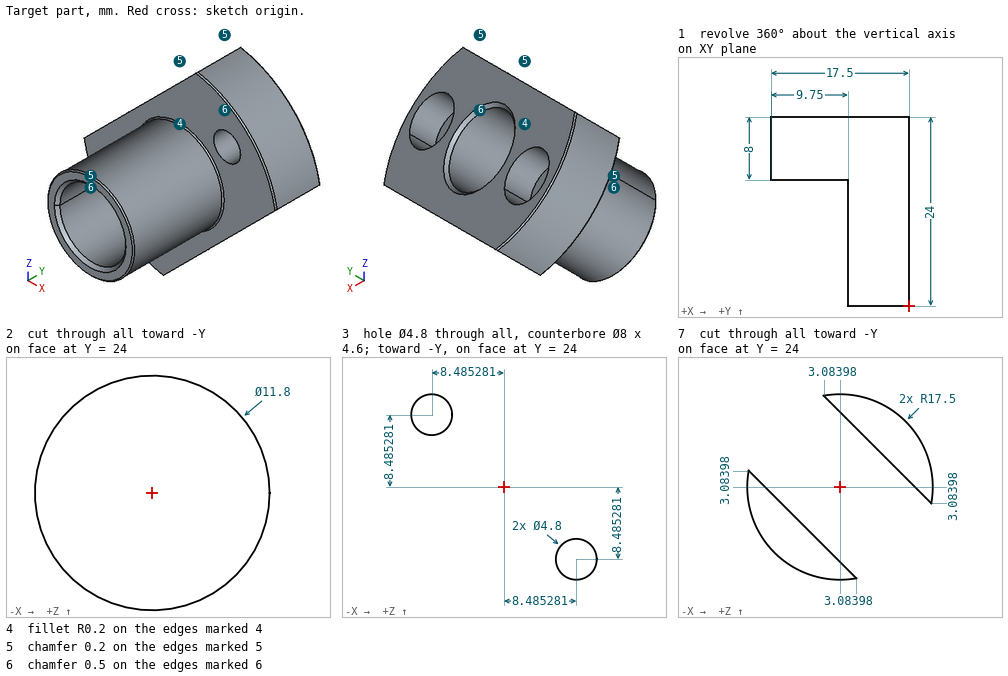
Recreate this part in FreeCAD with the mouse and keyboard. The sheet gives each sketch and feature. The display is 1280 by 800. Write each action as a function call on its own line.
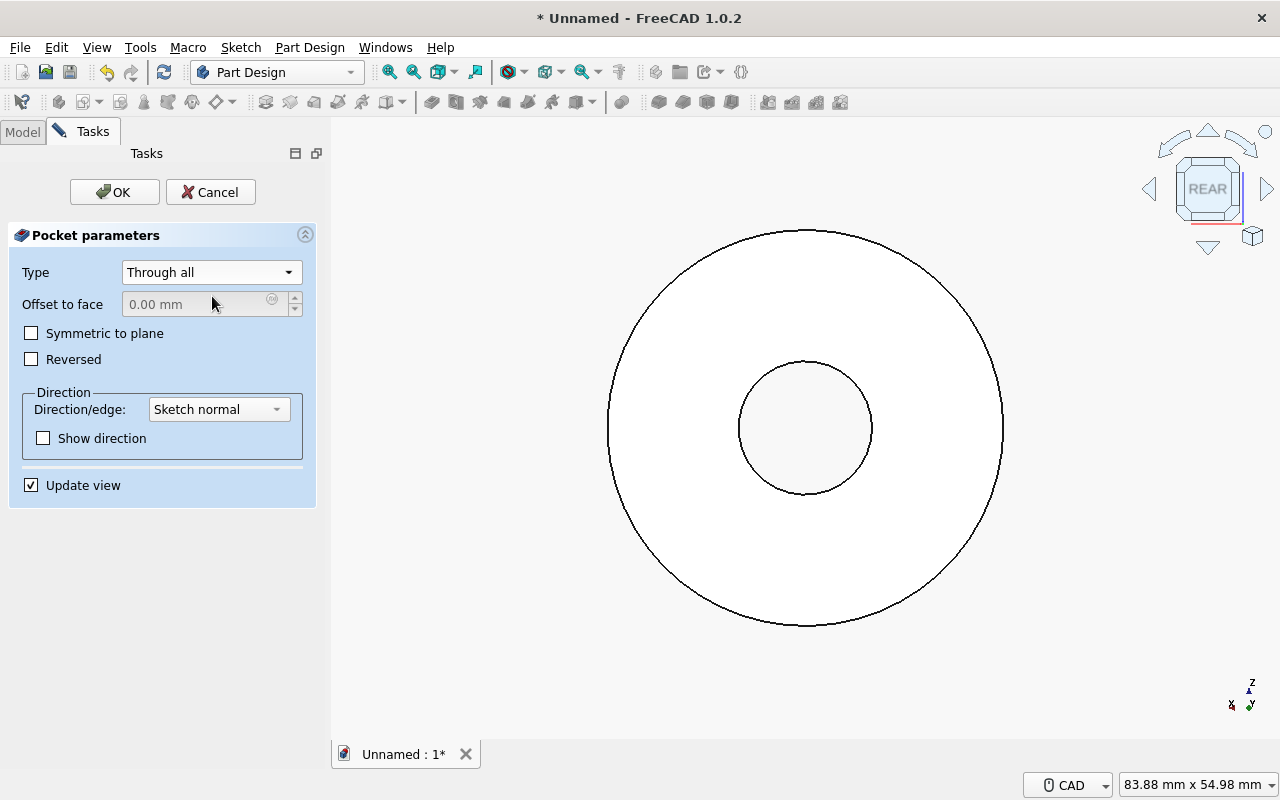
click(115, 192)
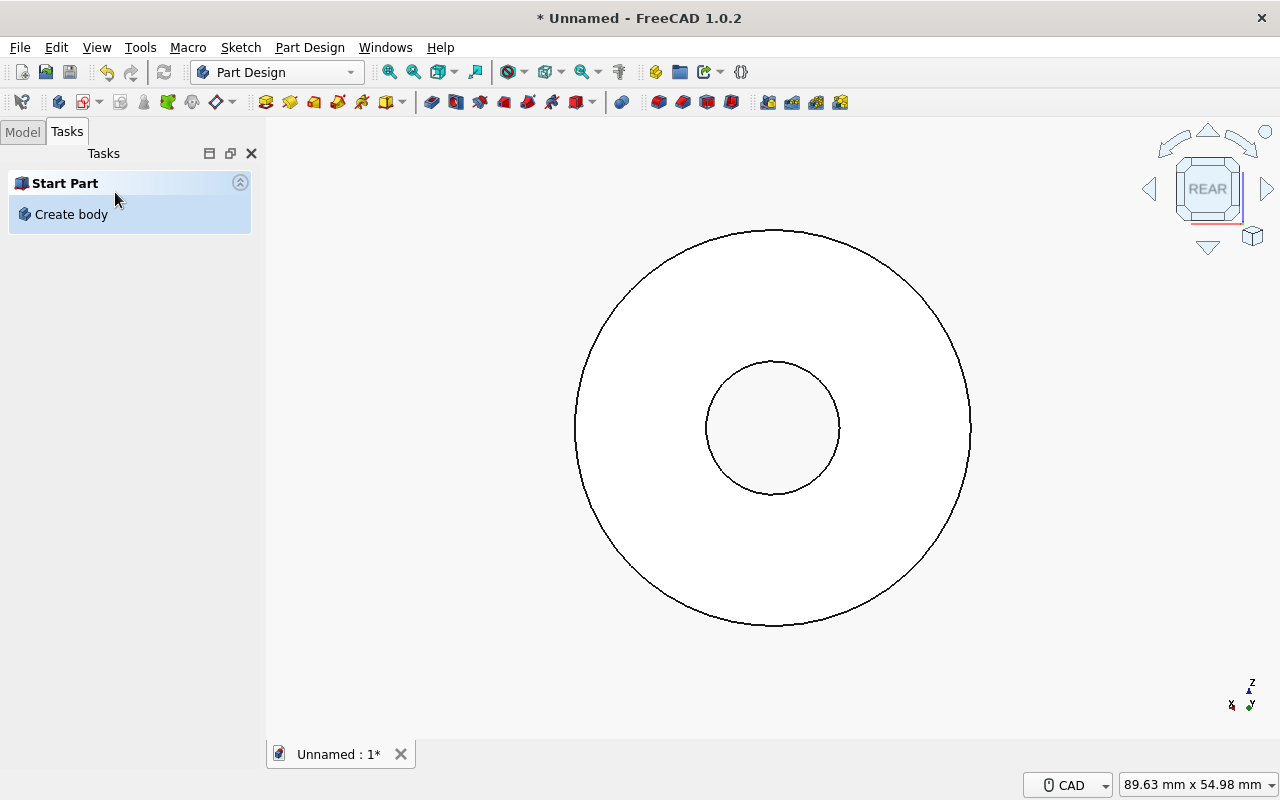
click(829, 540)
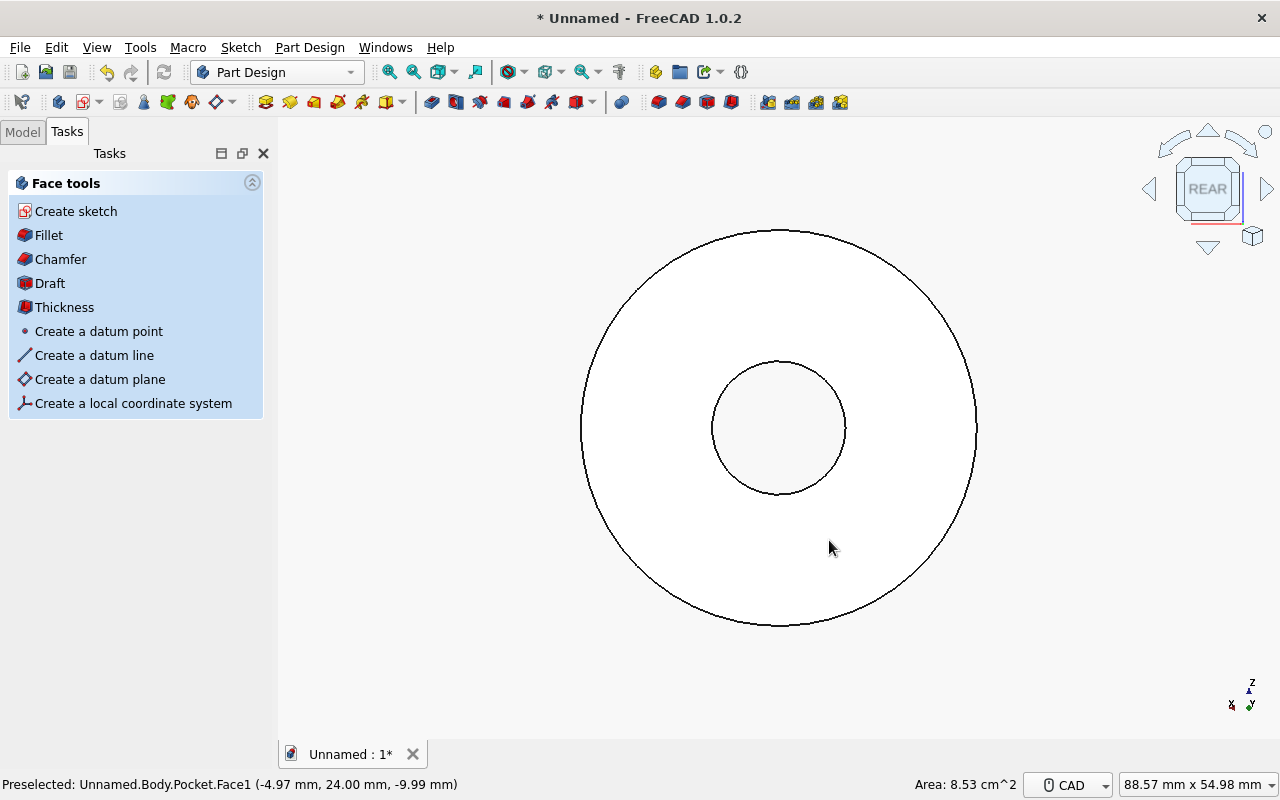
click(84, 102)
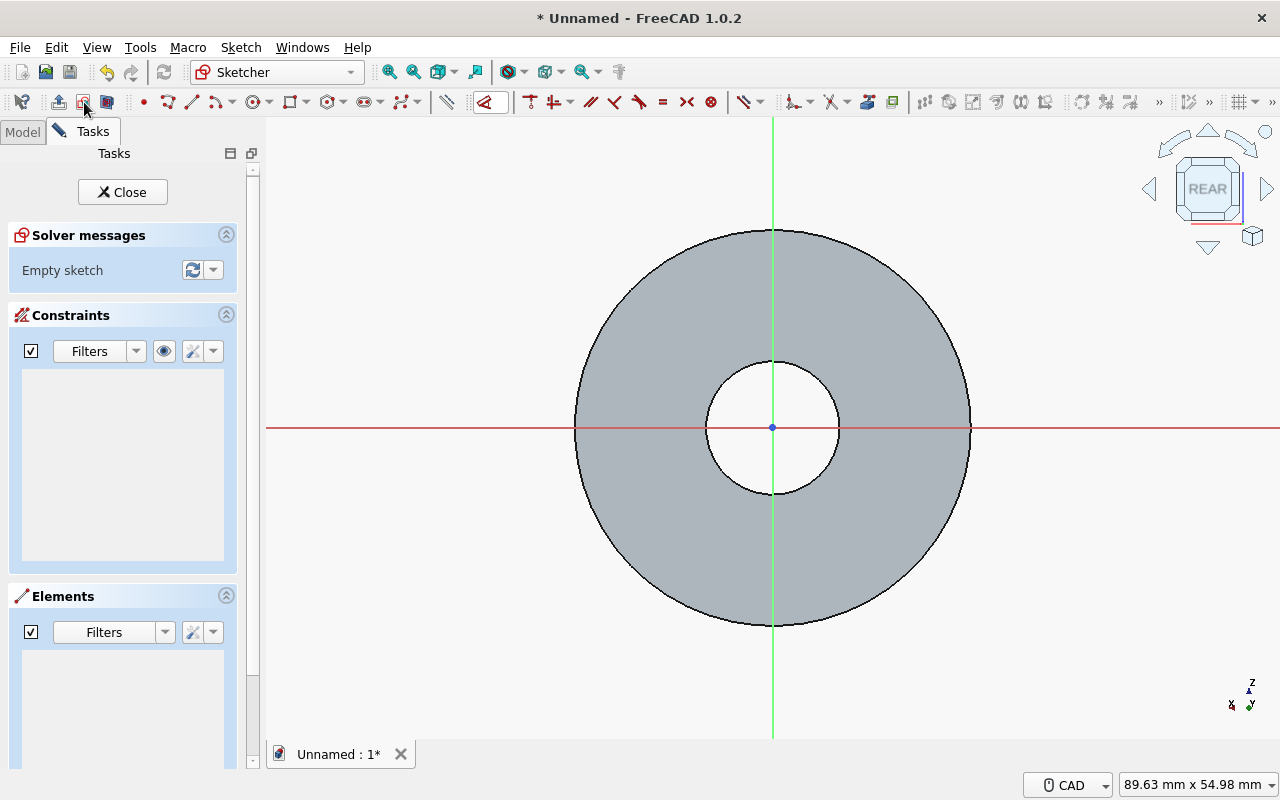
scroll(912, 428, up, 2)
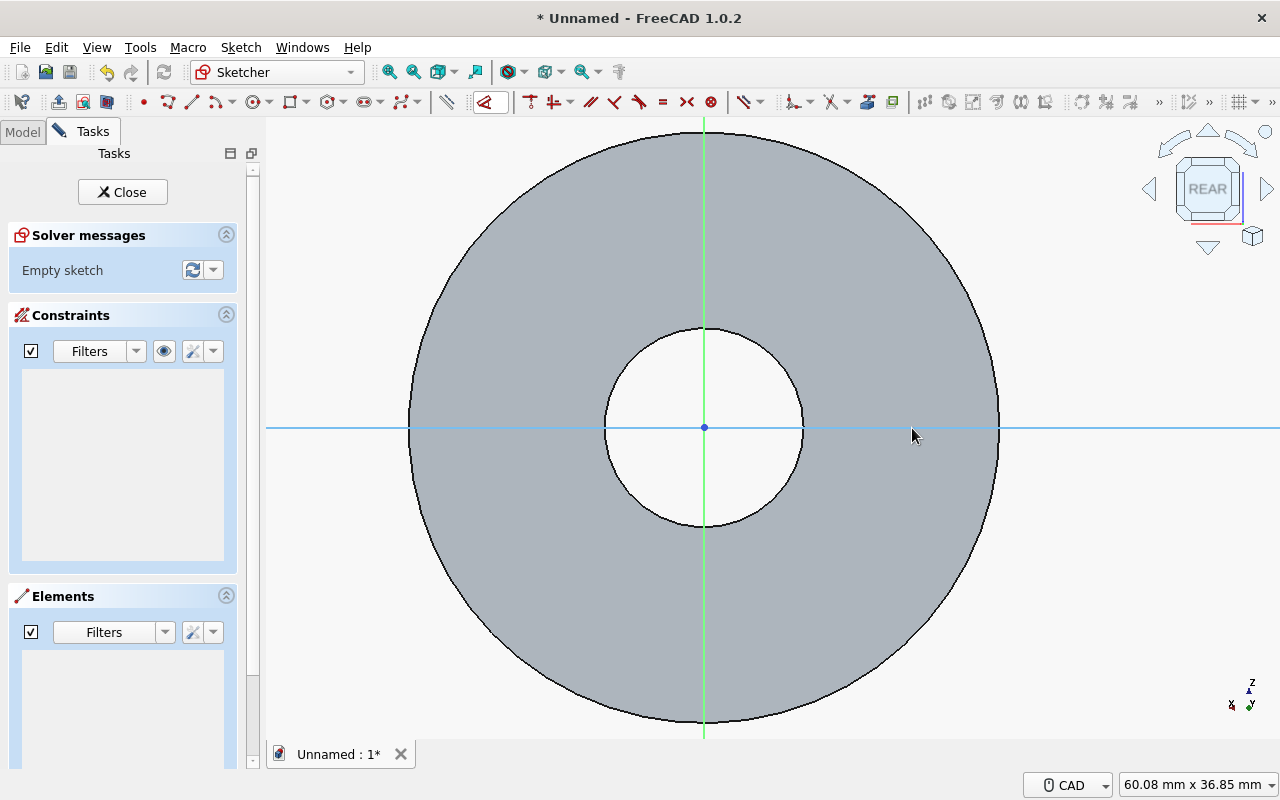
key(g)
key(c)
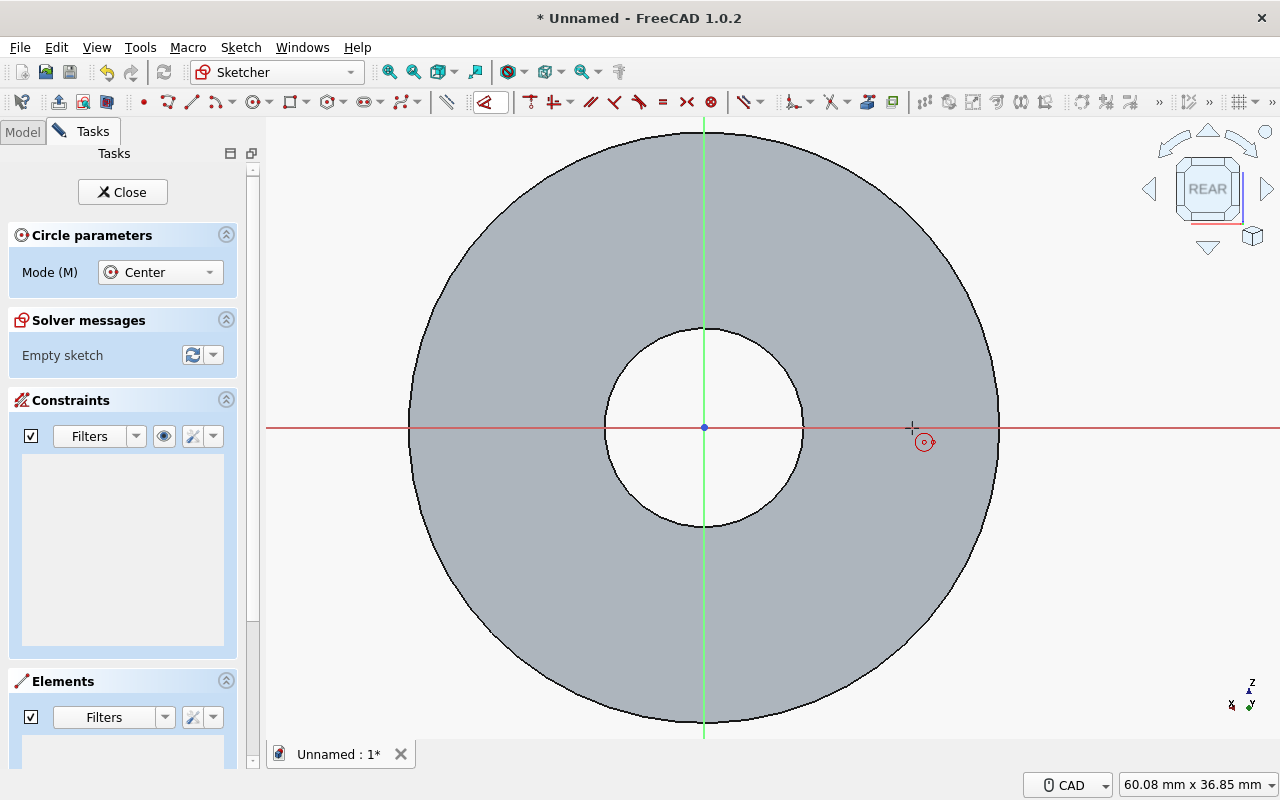
click(847, 571)
click(876, 542)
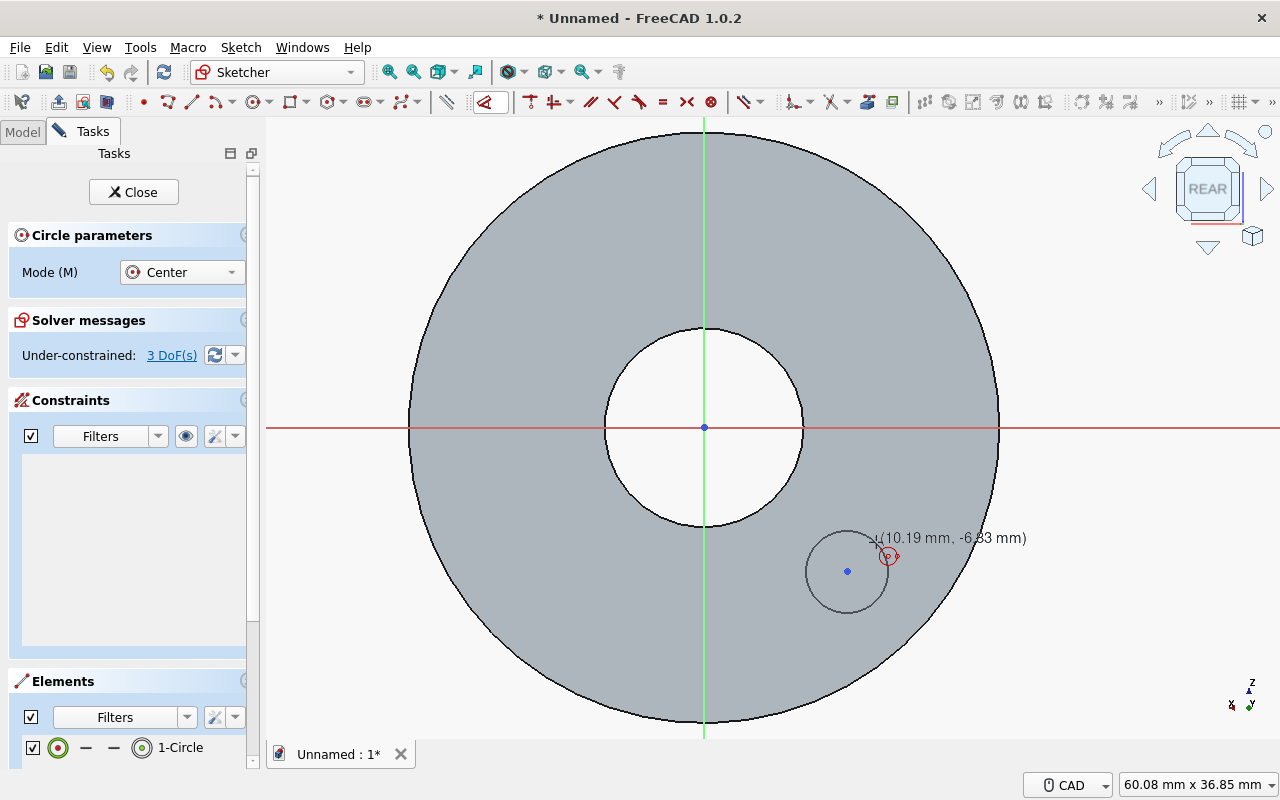
click(561, 285)
click(589, 256)
key(Escape)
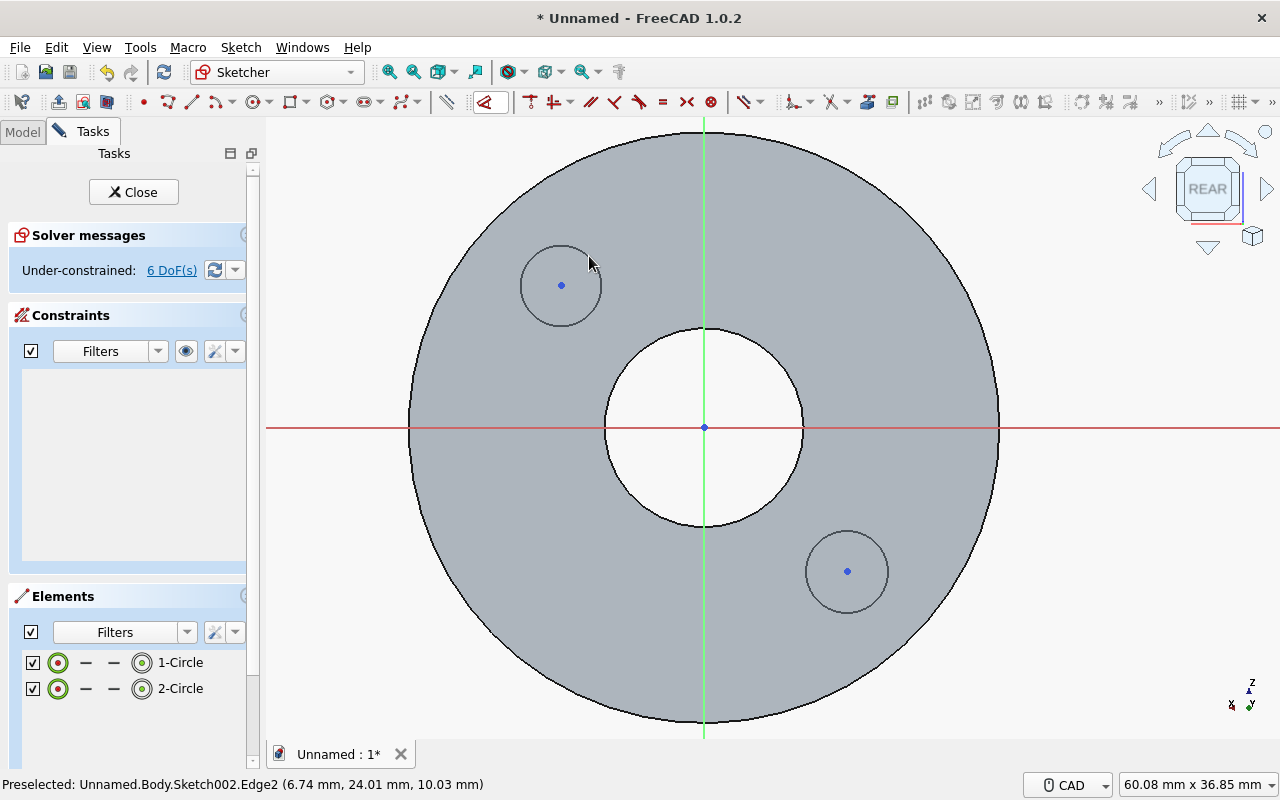
click(876, 543)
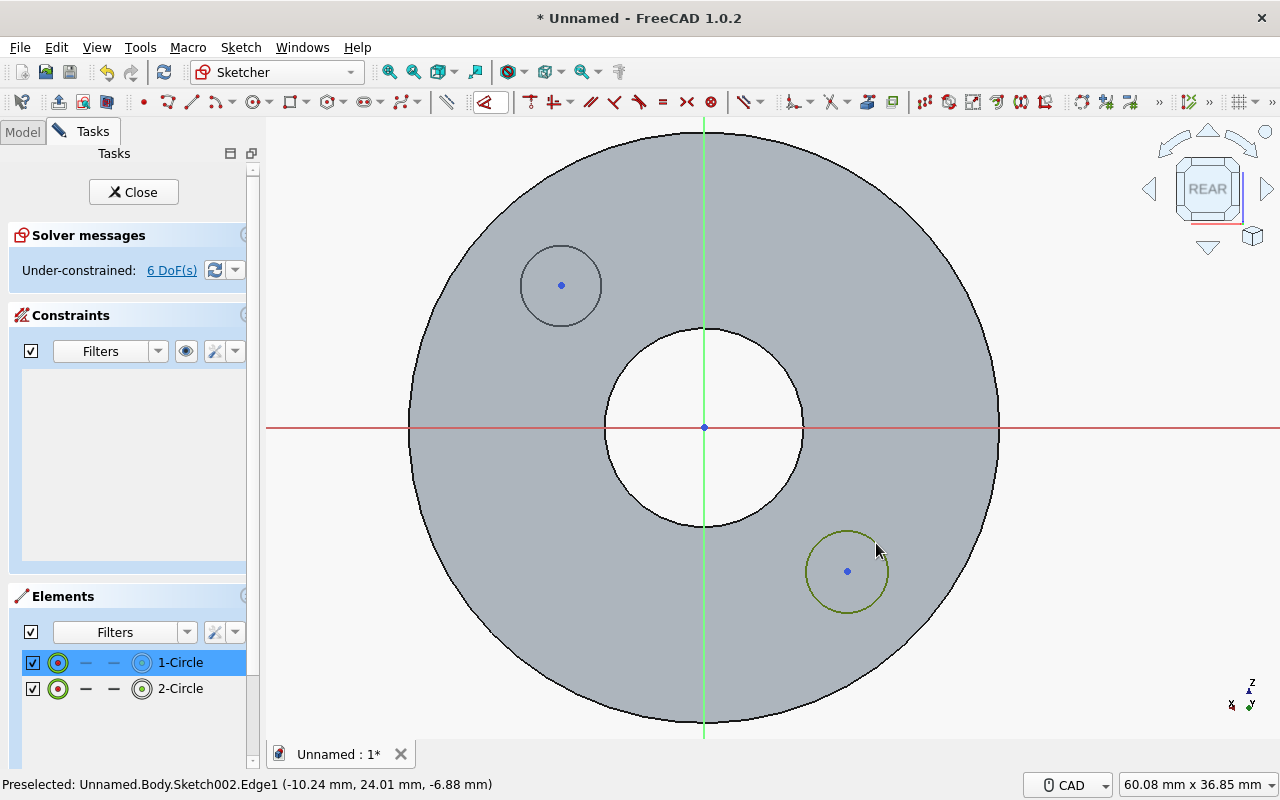
click(589, 257)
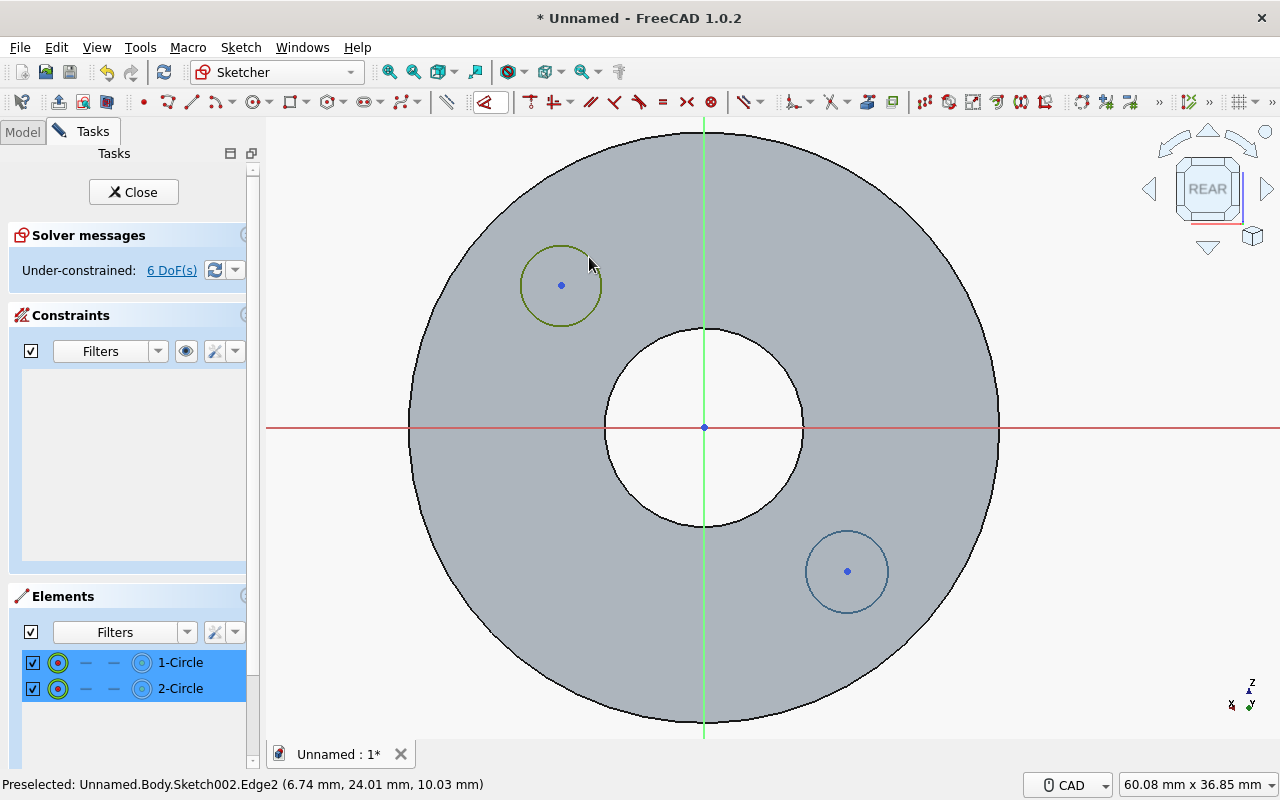
key(e)